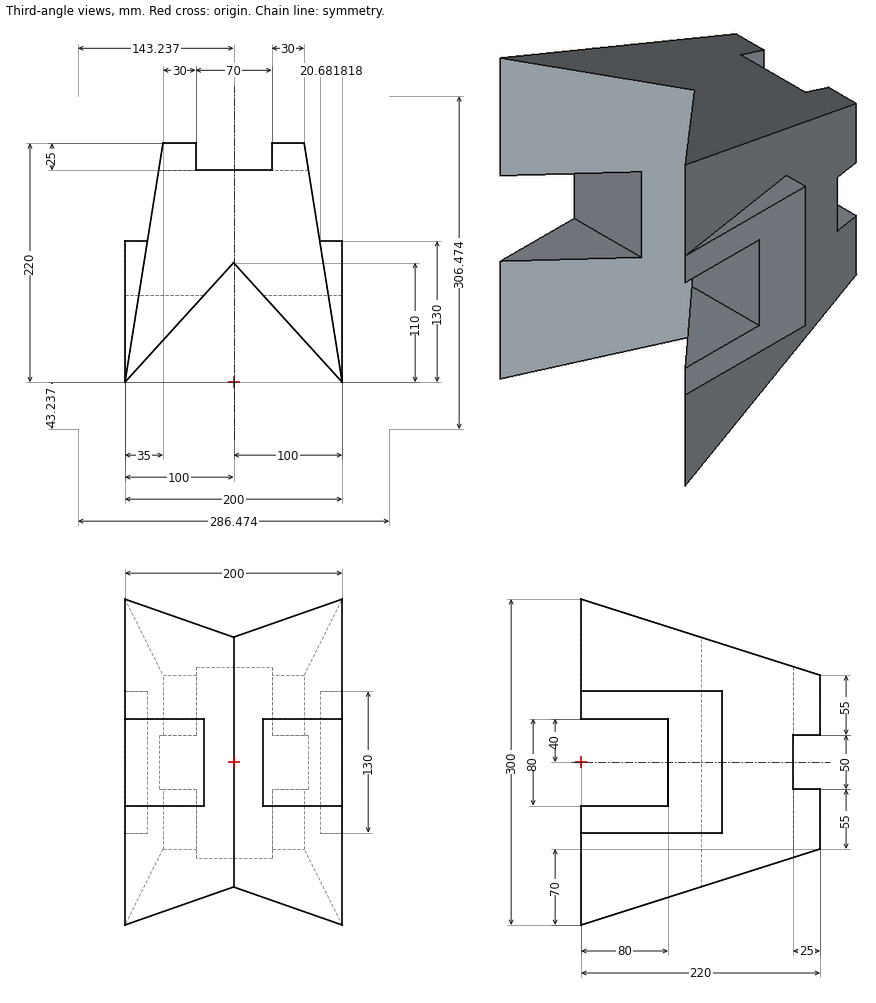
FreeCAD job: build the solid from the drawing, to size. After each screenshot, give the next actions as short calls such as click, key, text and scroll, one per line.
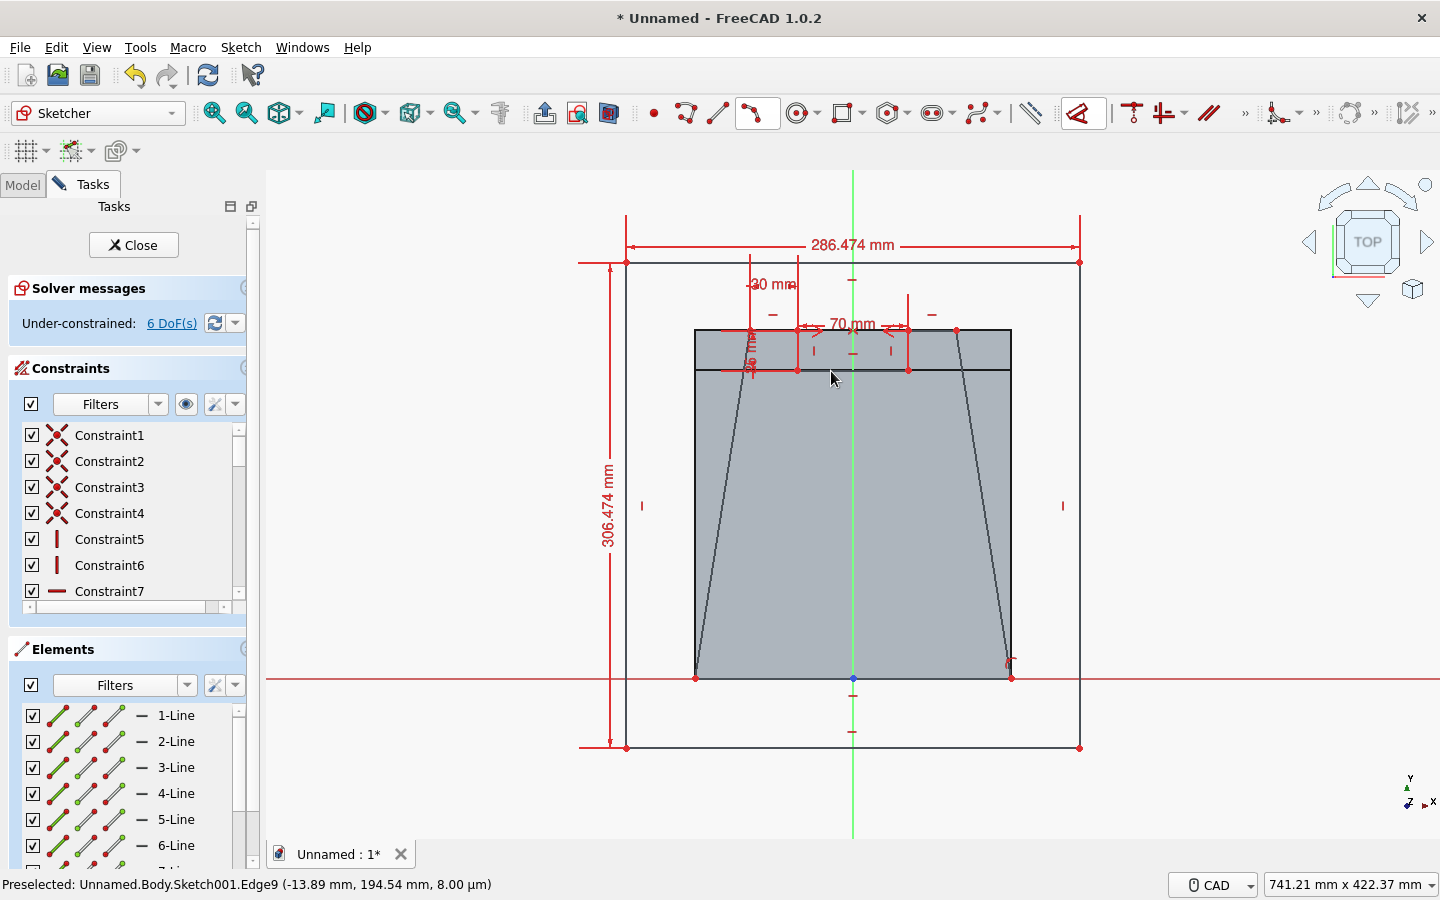
click(923, 331)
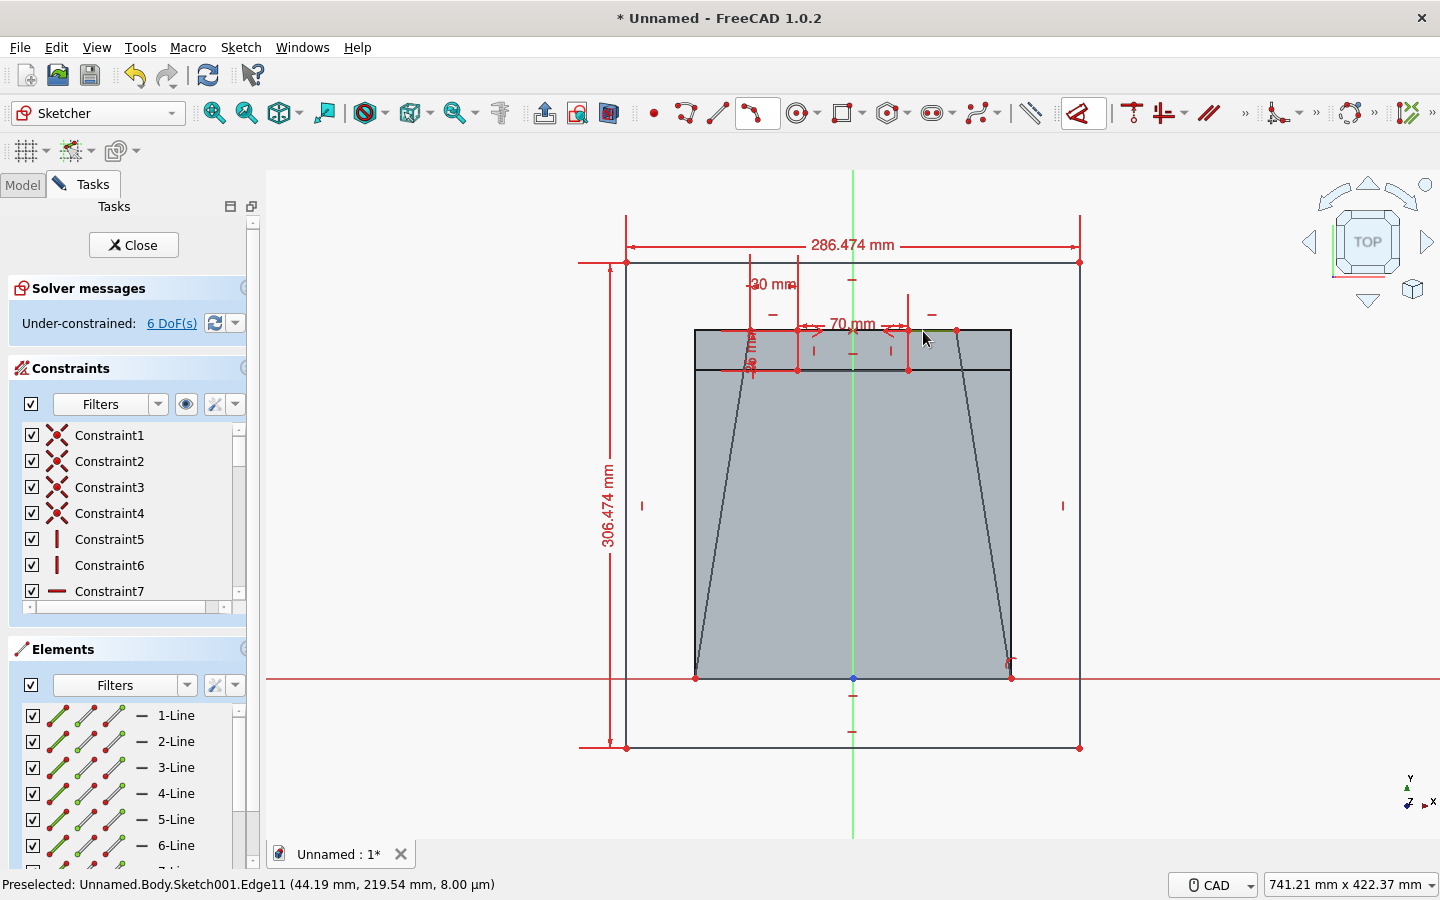
key(l)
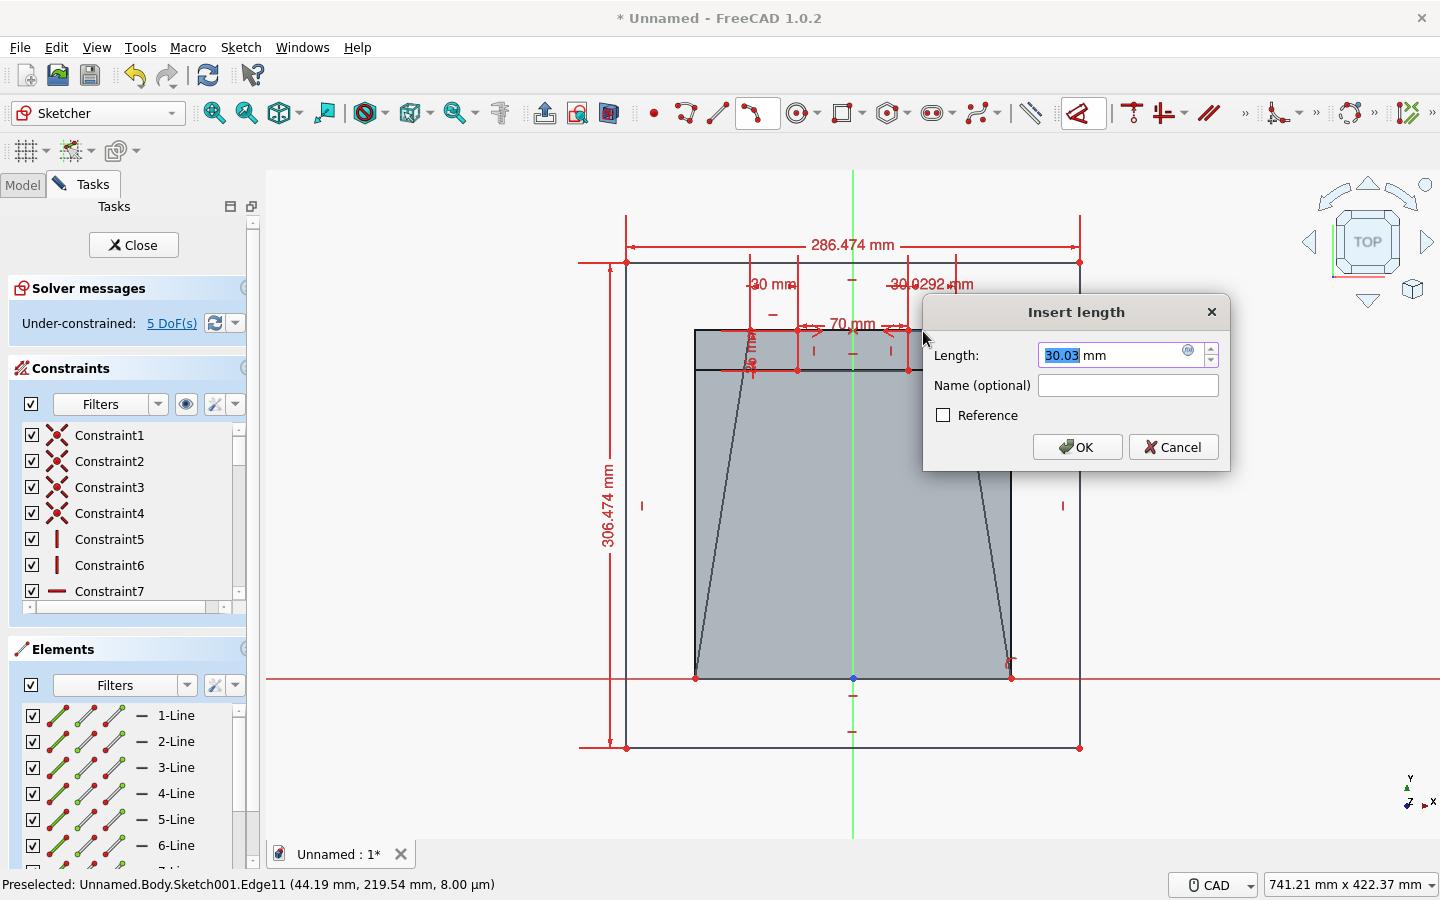
text(30)
key(Return)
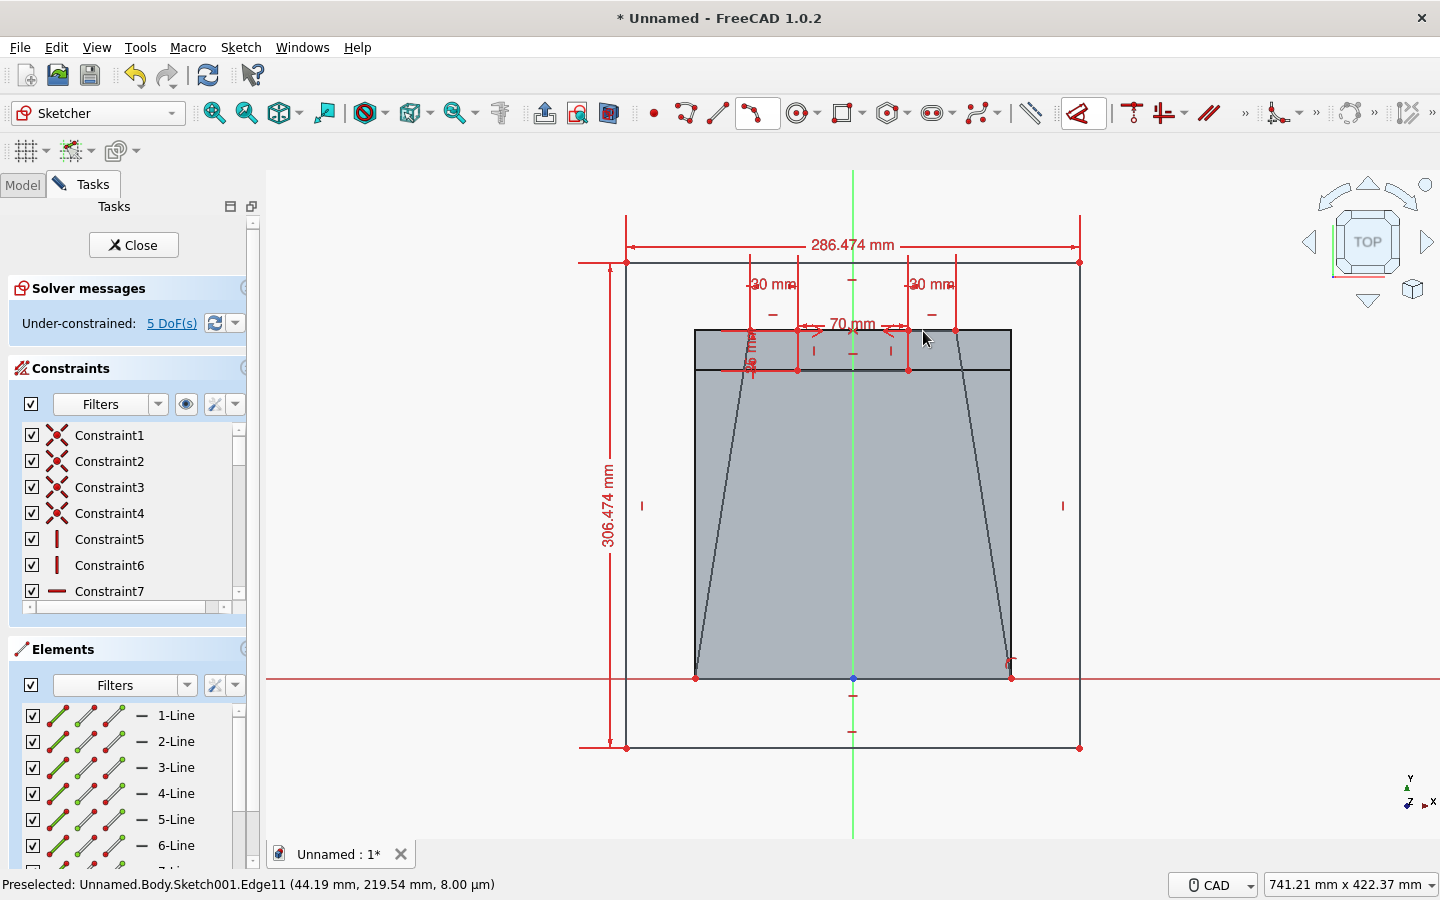
click(916, 679)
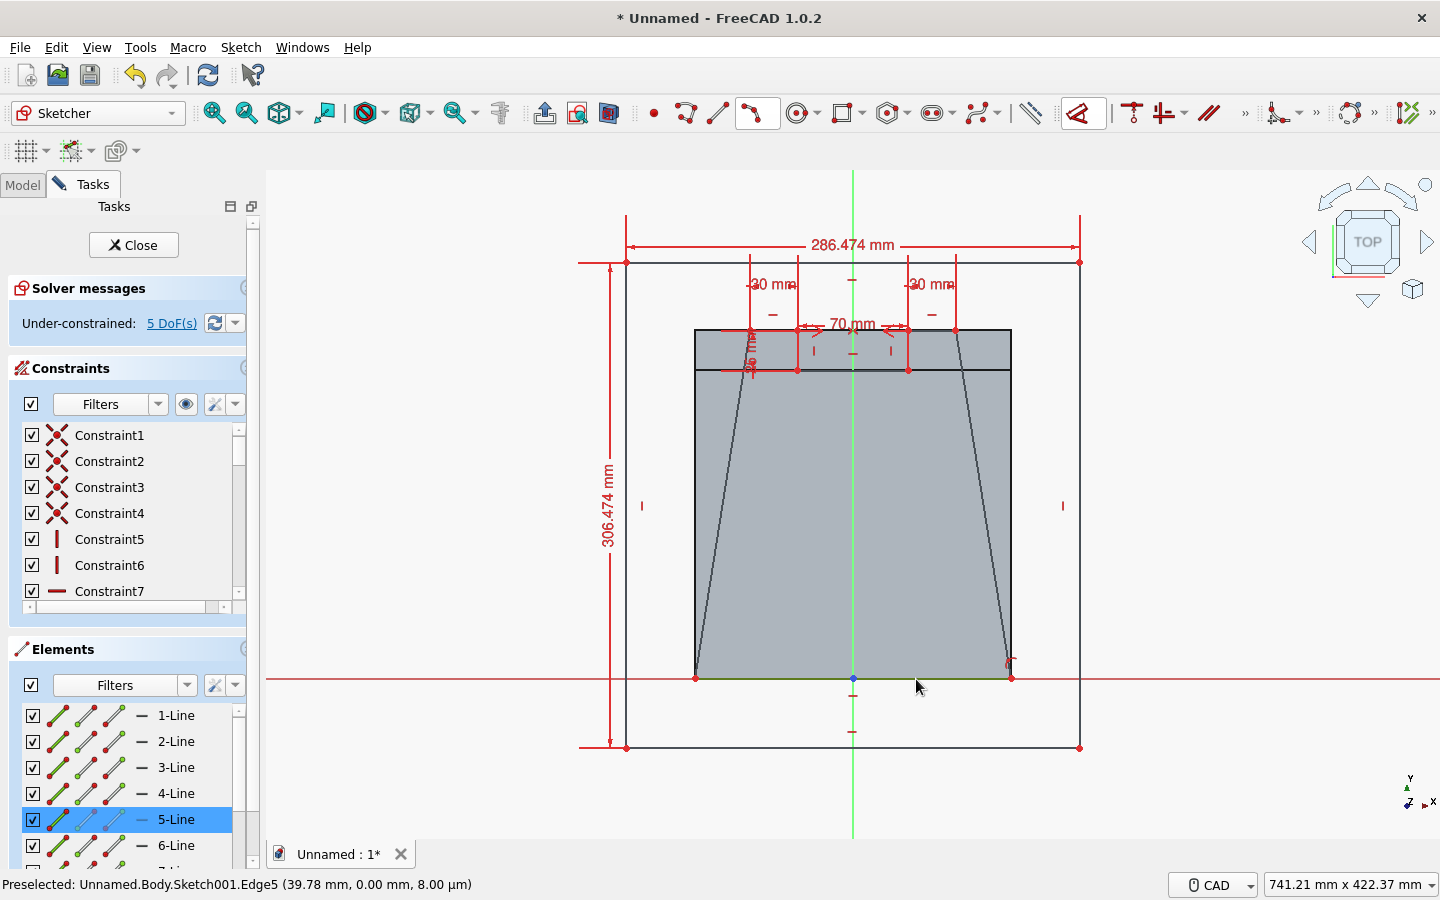
key(l)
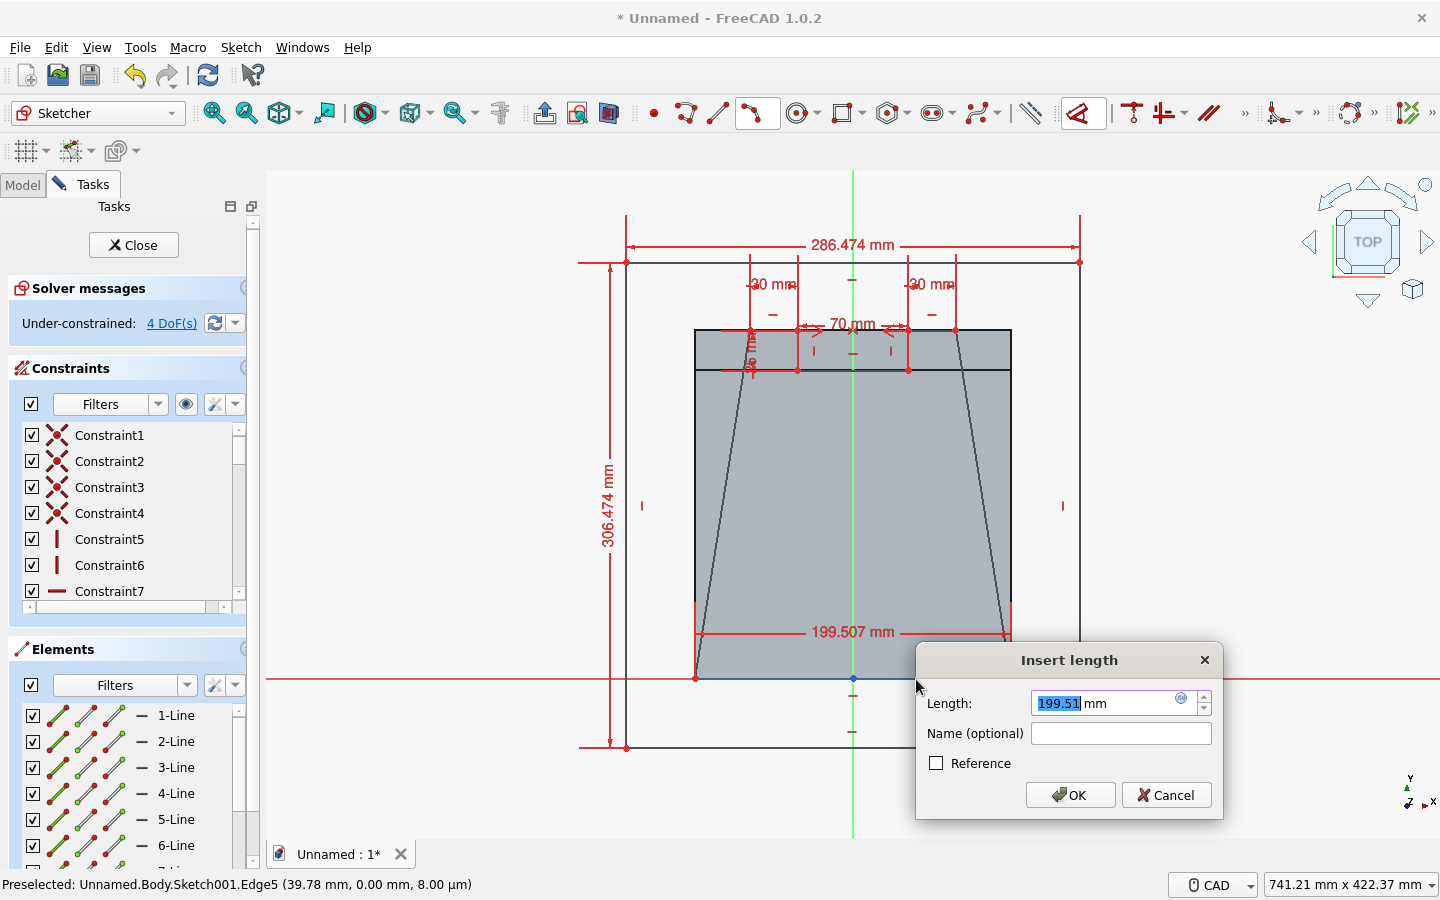
text(200)
key(Return)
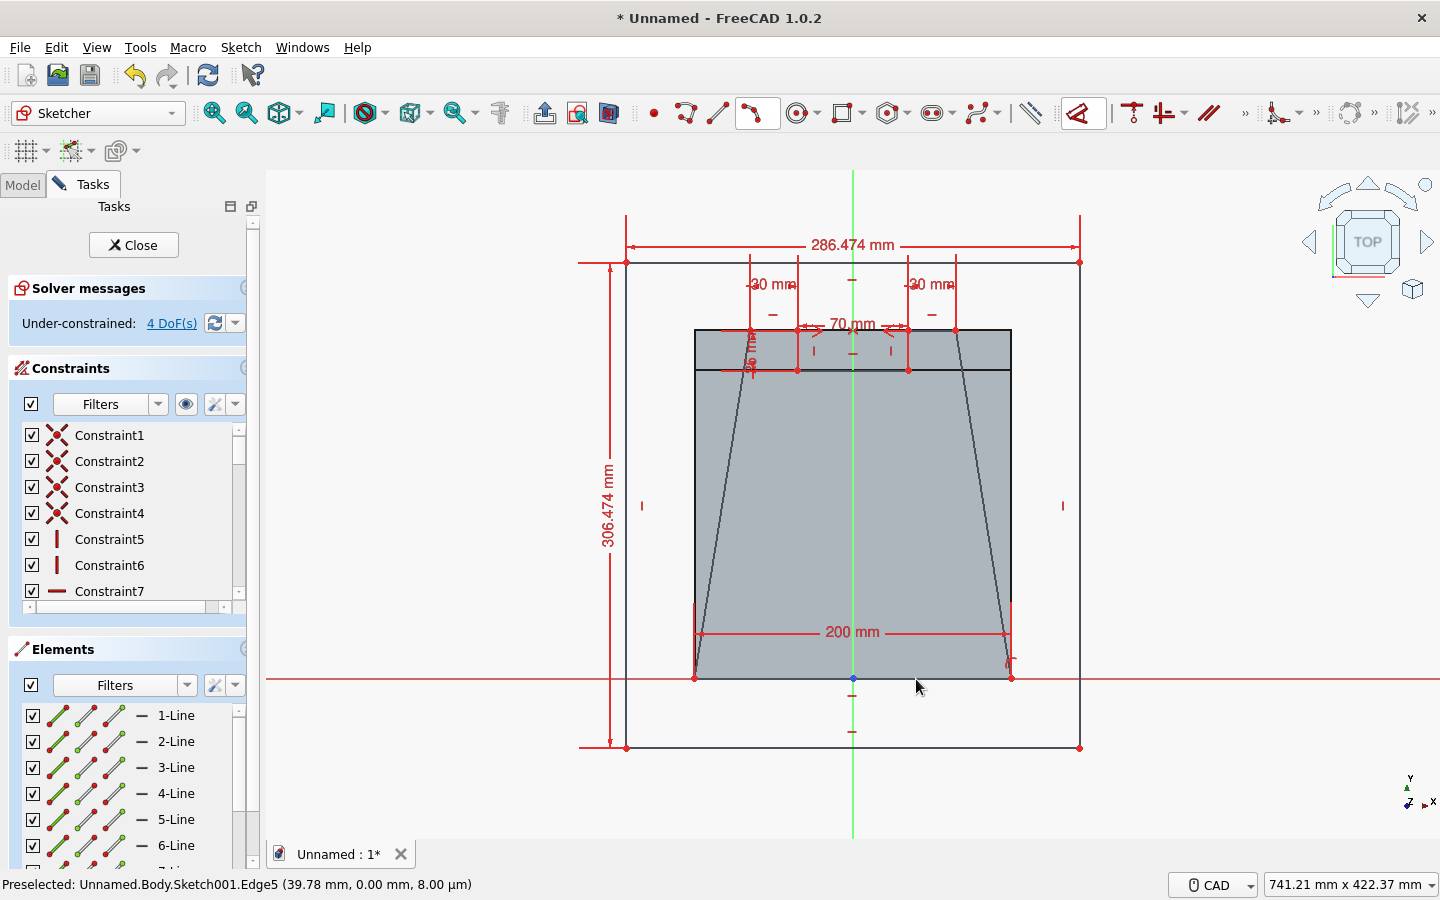
click(711, 574)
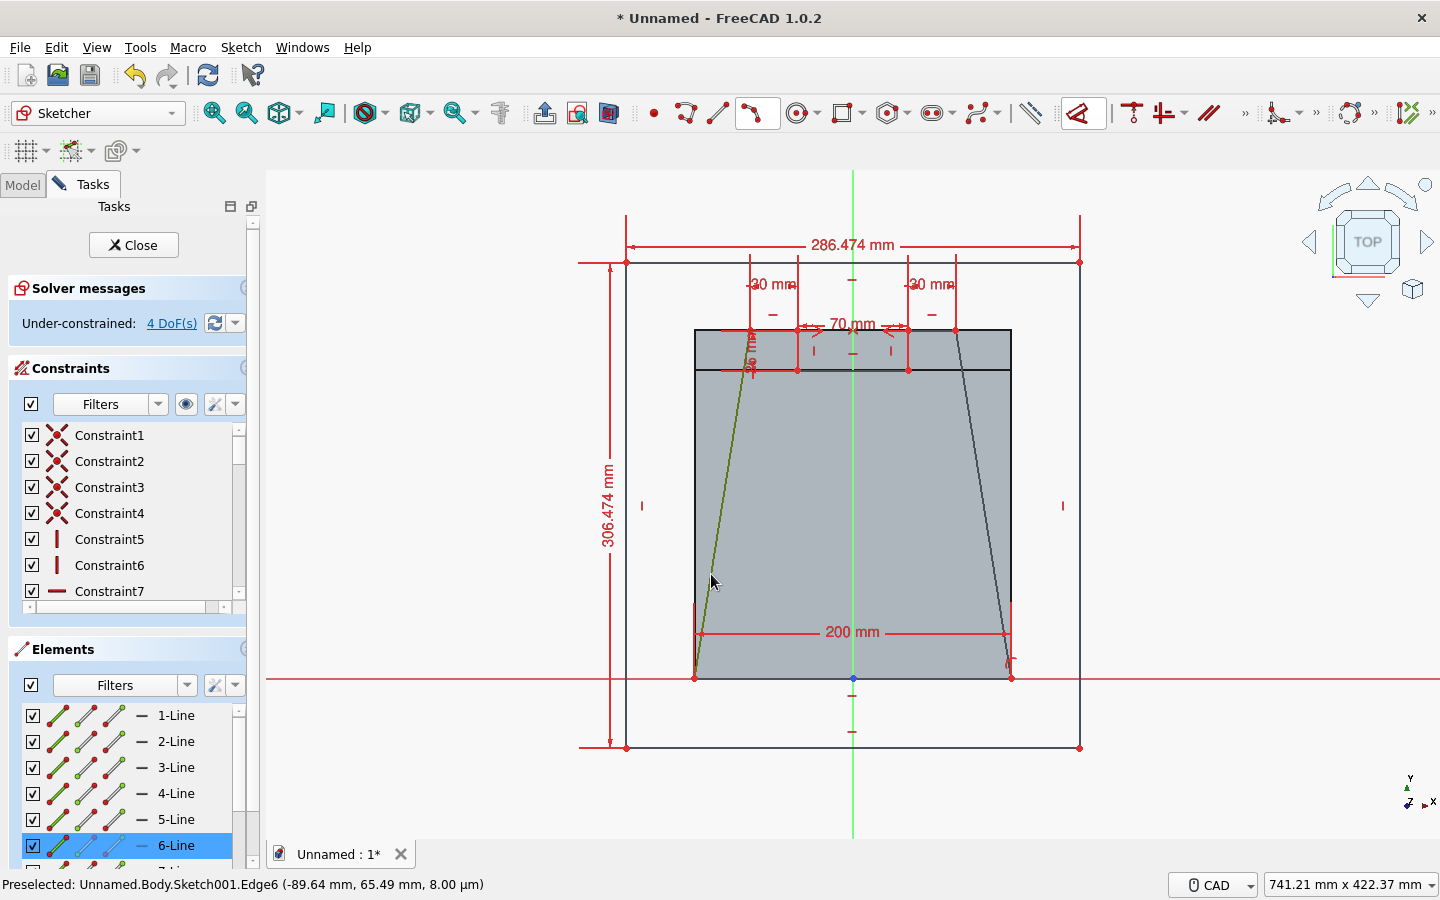
key(l)